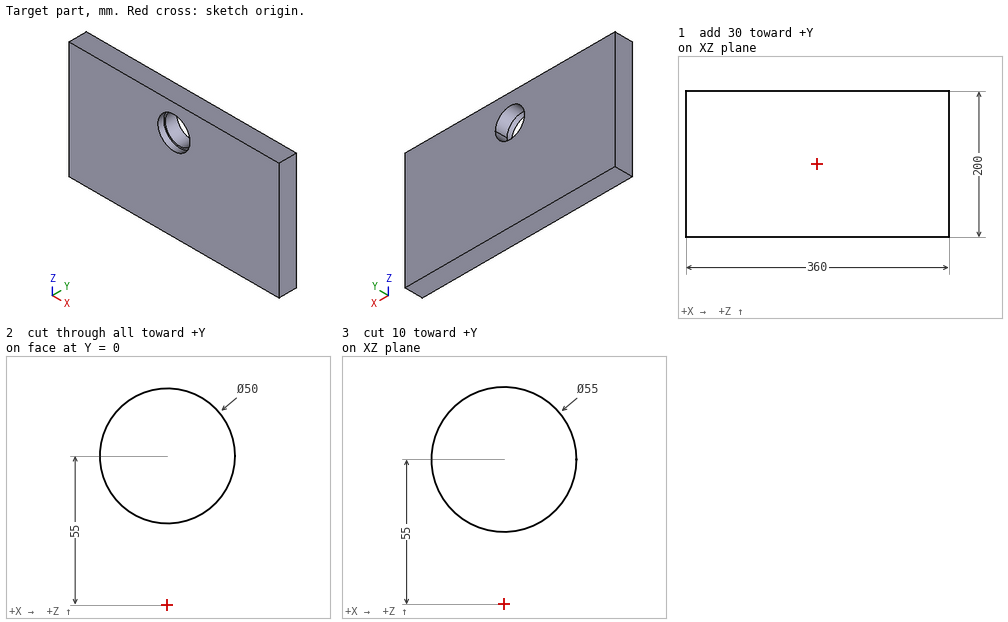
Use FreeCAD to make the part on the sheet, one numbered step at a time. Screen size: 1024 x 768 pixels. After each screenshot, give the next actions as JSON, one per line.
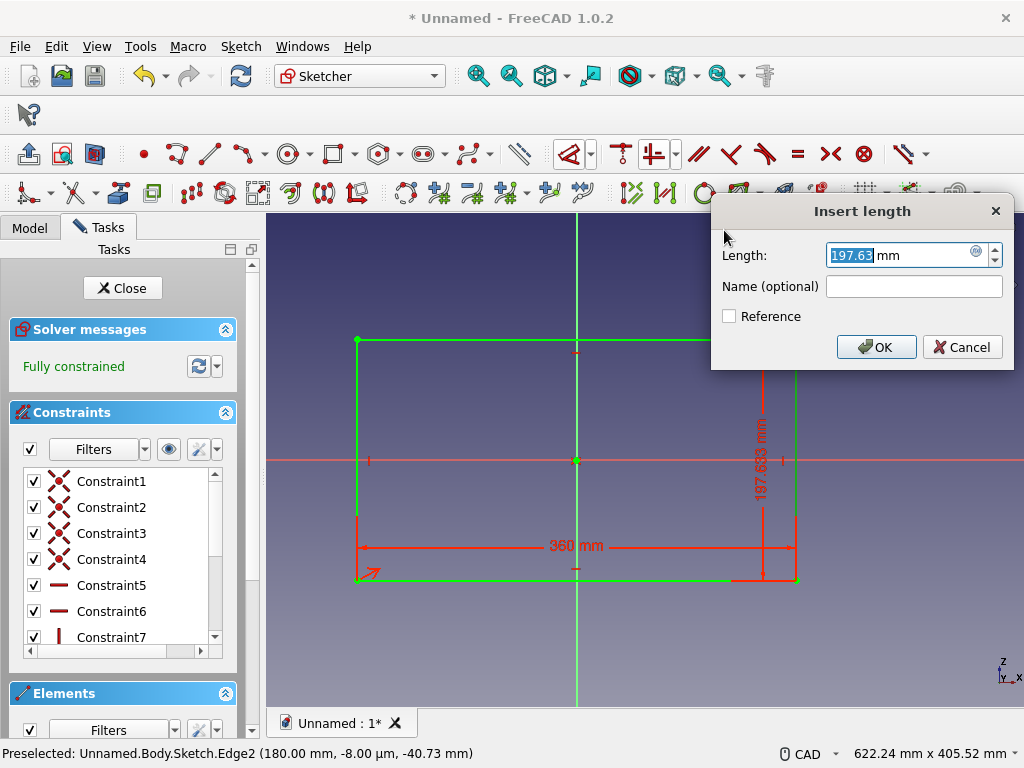
{"action": "type", "text": "200"}
{"action": "key", "text": "Return"}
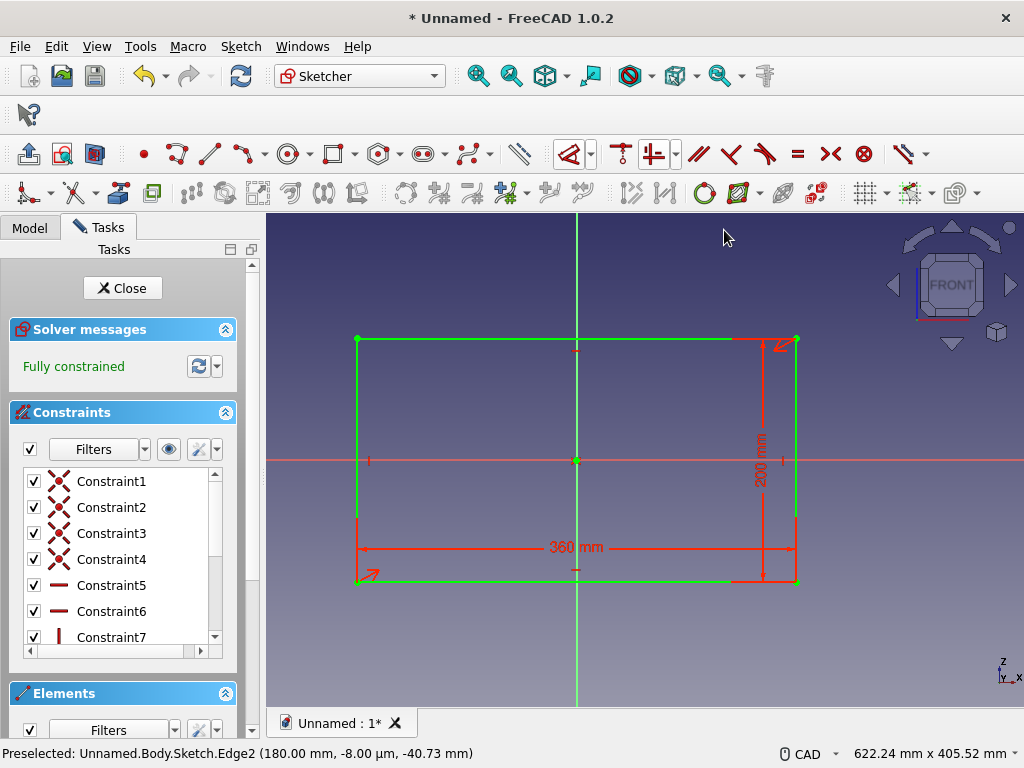
{"action": "left_click", "coordinate": [123, 288]}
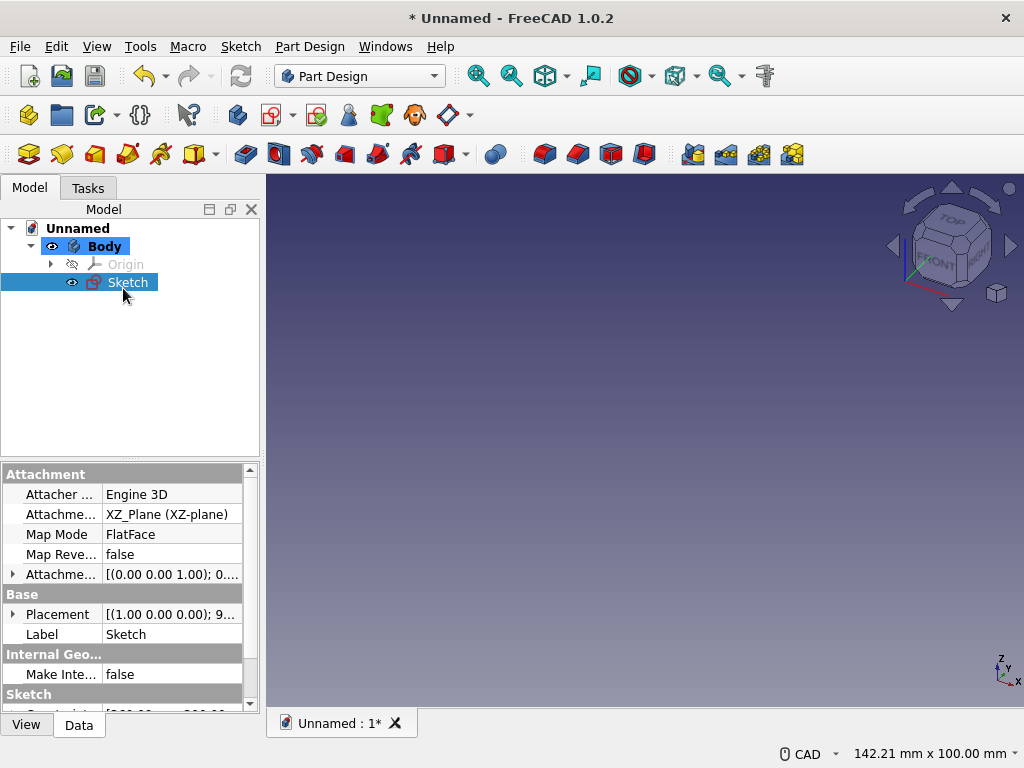
{"action": "left_click", "coordinate": [29, 154]}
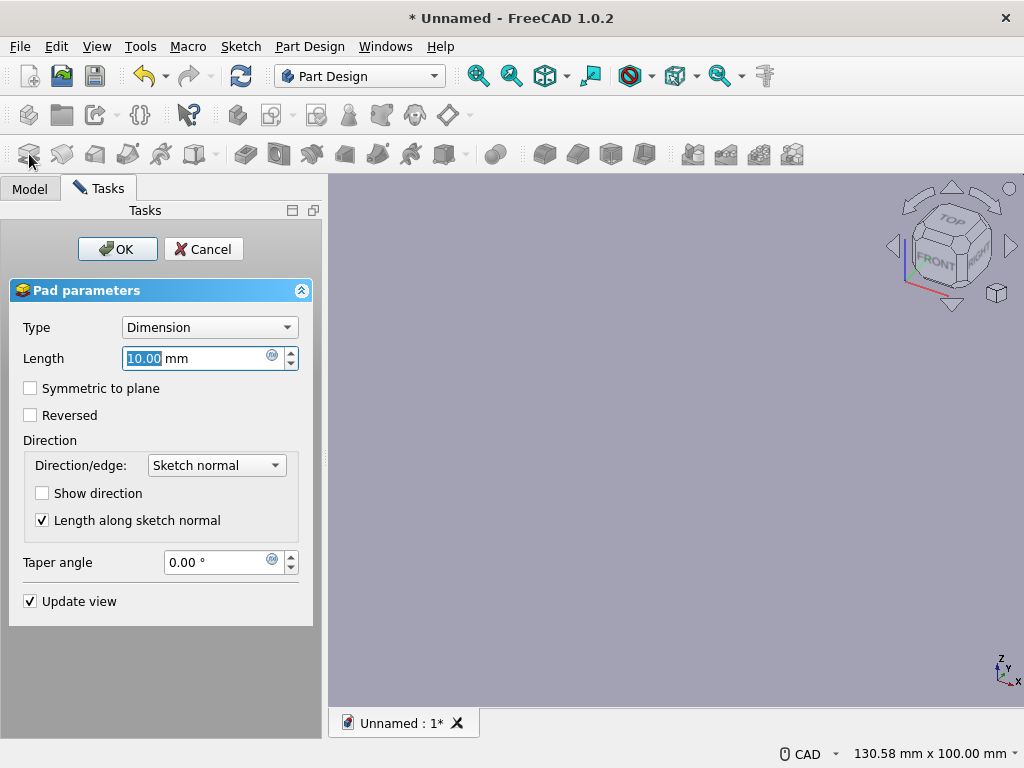
{"action": "type", "text": "30"}
{"action": "key", "text": "Tab"}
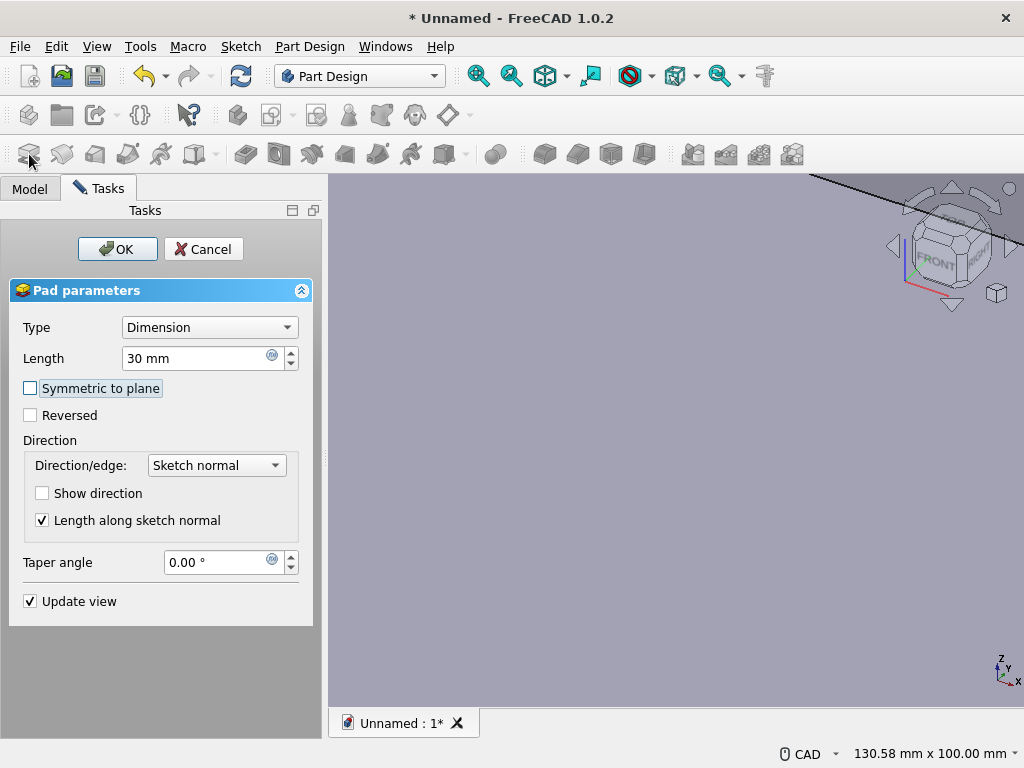
{"action": "left_click", "coordinate": [31, 415]}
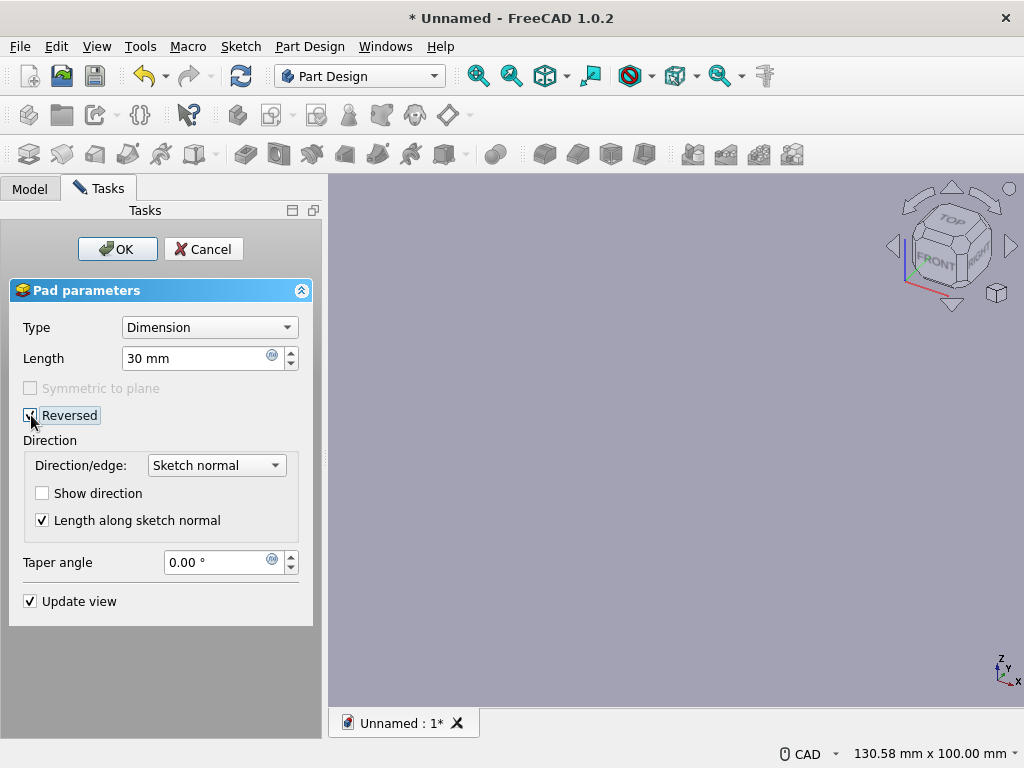
{"action": "left_click", "coordinate": [118, 249]}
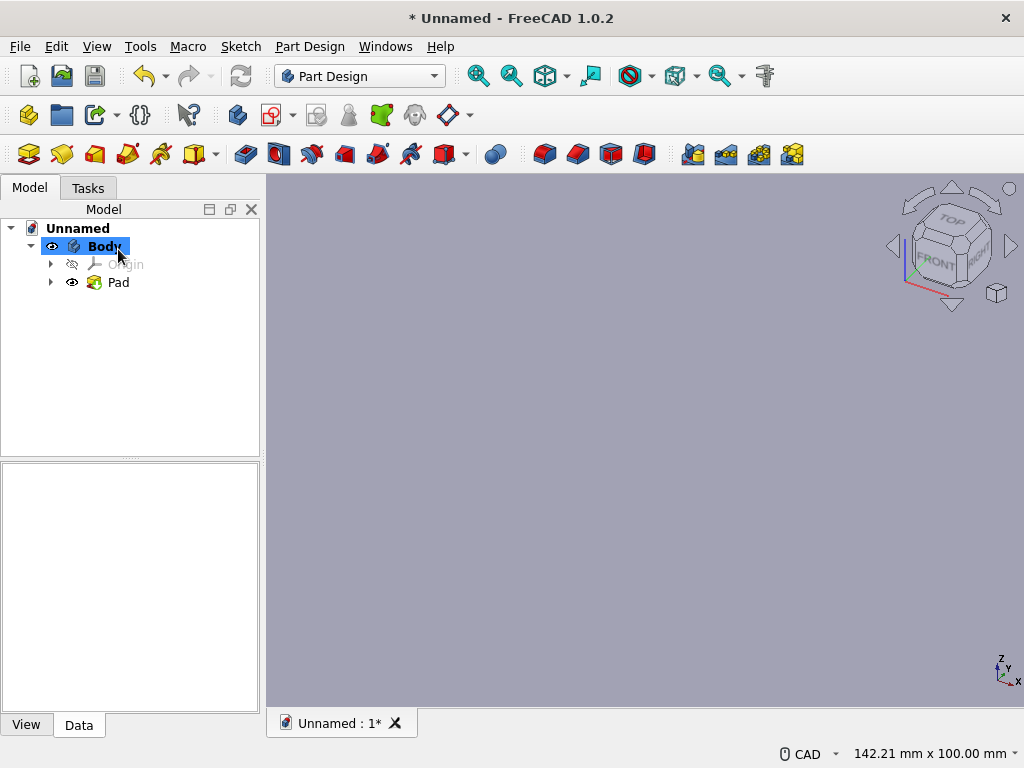
{"action": "key", "text": "v f"}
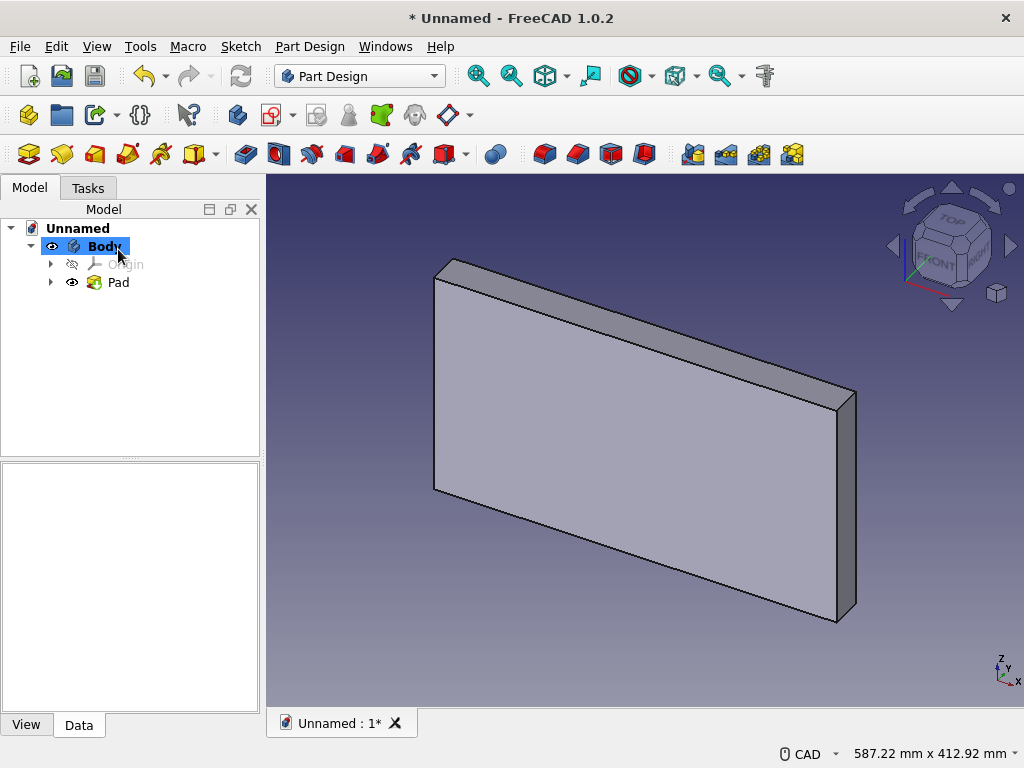
{"action": "left_click", "coordinate": [693, 468]}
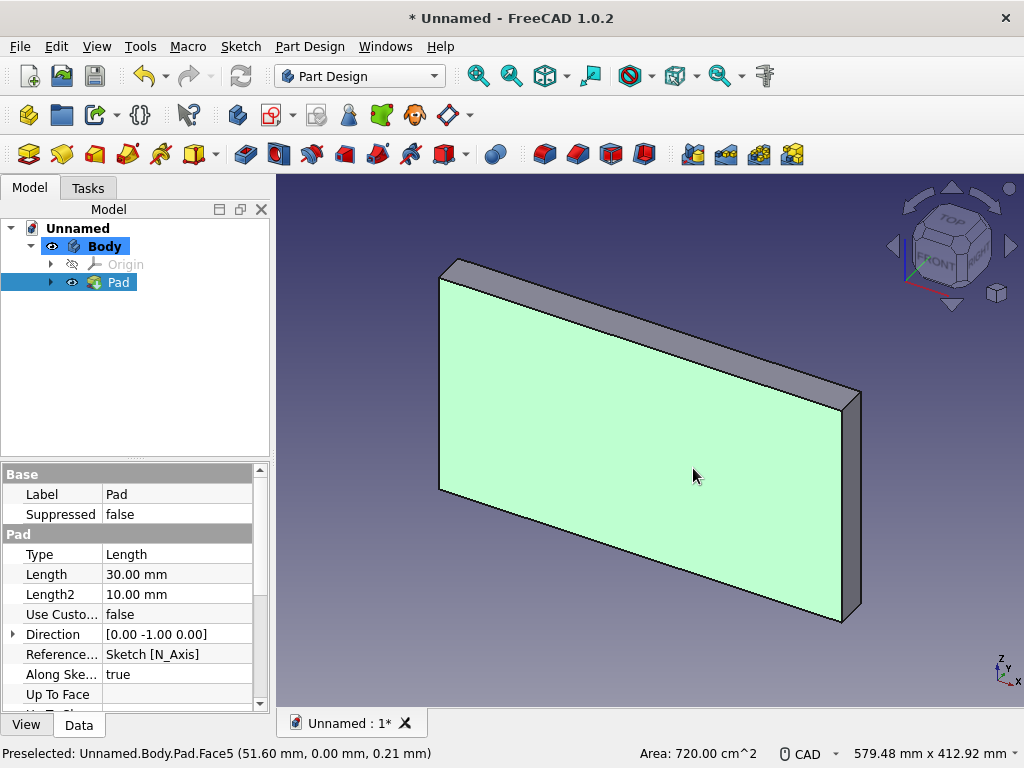
{"action": "left_click", "coordinate": [270, 116]}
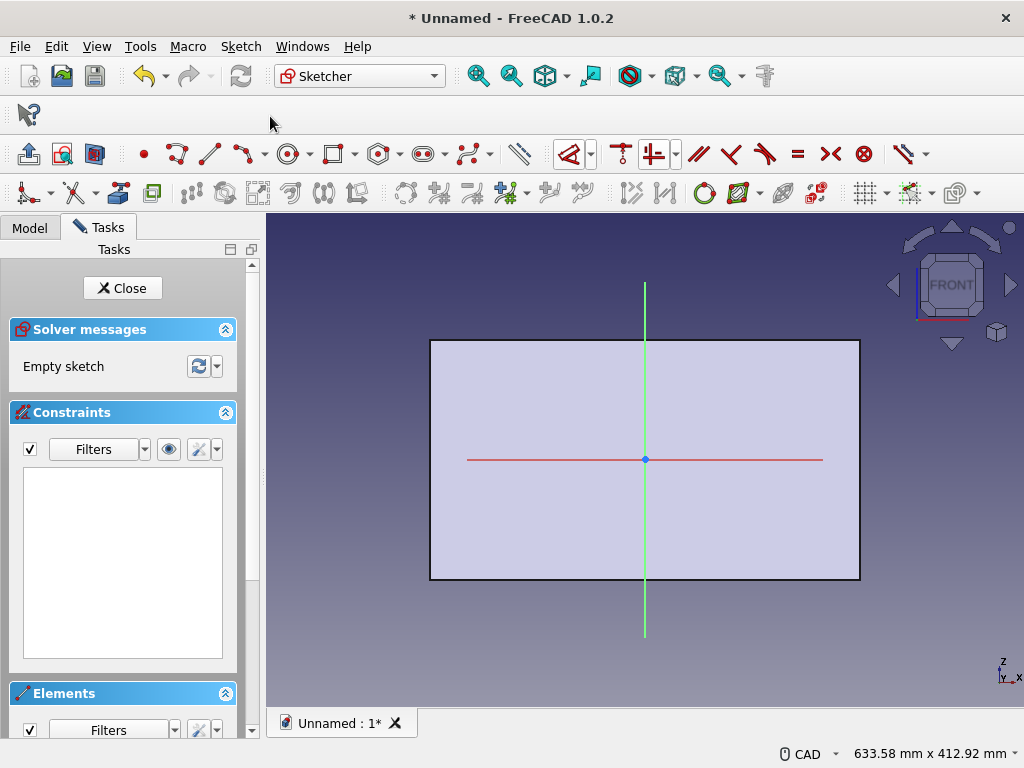
{"action": "scroll", "coordinate": [675, 392], "scroll_direction": "up", "scroll_amount": 6}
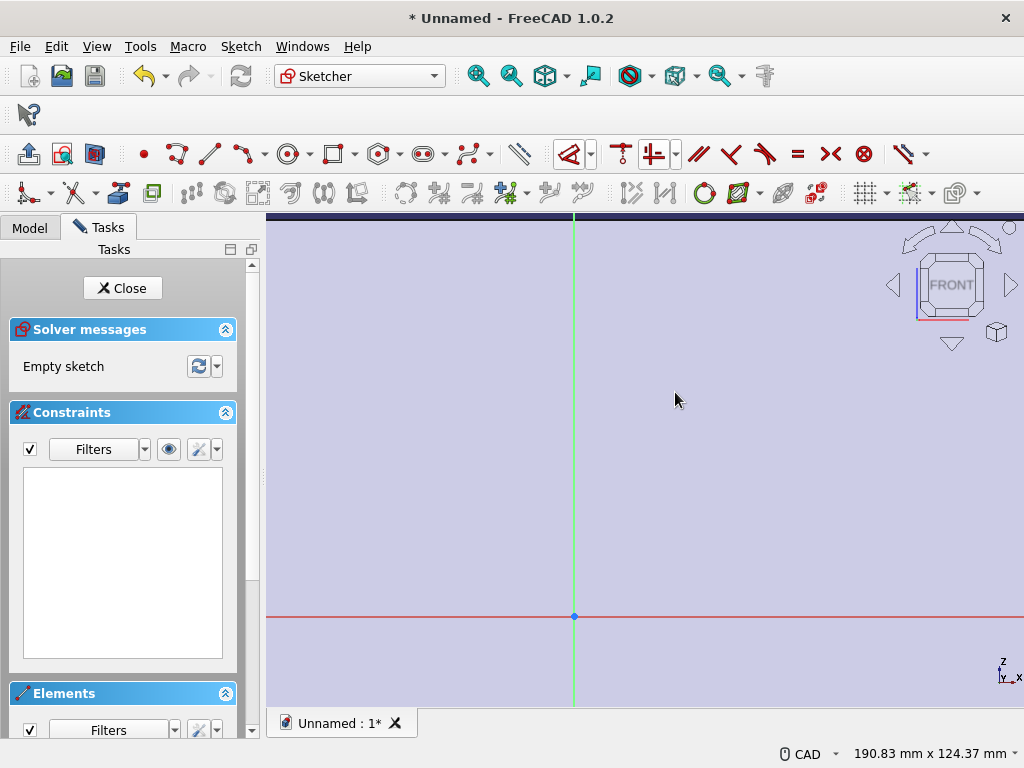
{"action": "left_click", "coordinate": [288, 154]}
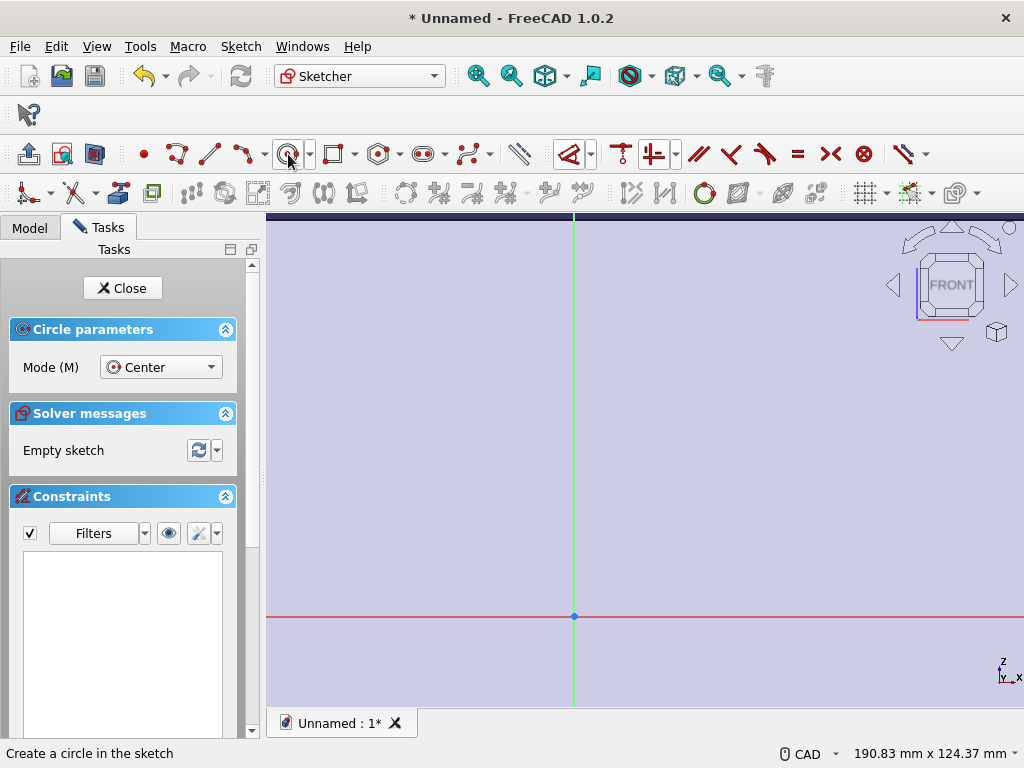
{"action": "left_click", "coordinate": [574, 398]}
{"action": "left_click", "coordinate": [644, 328]}
{"action": "key", "text": "Escape"}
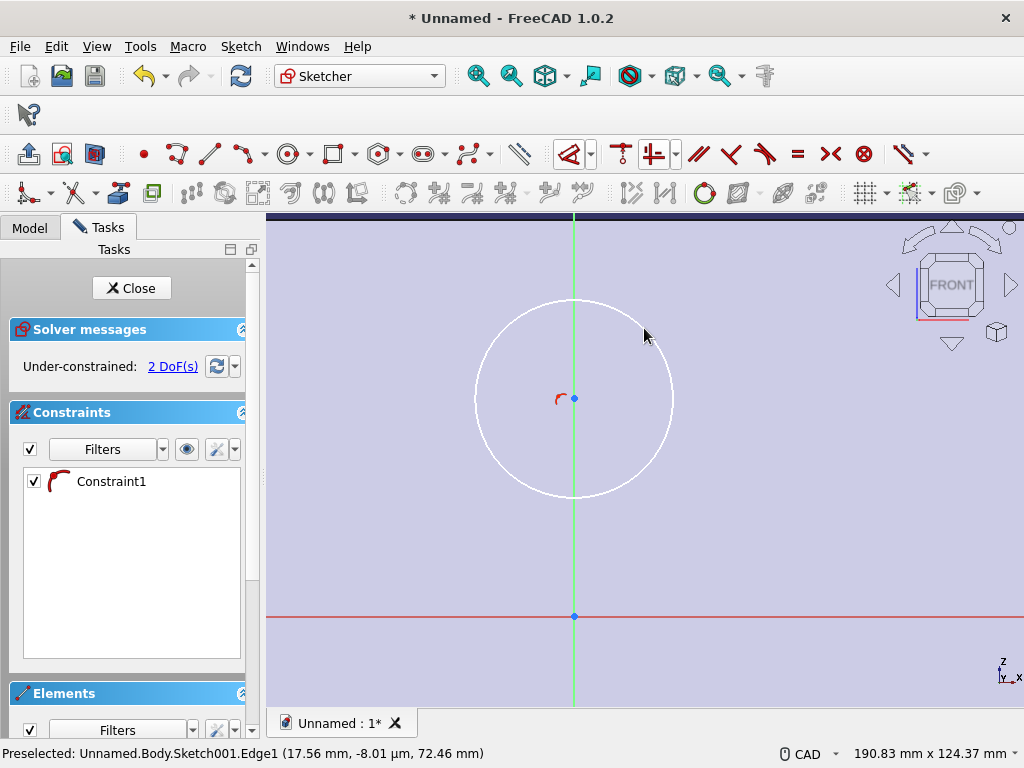
{"action": "left_click", "coordinate": [644, 329]}